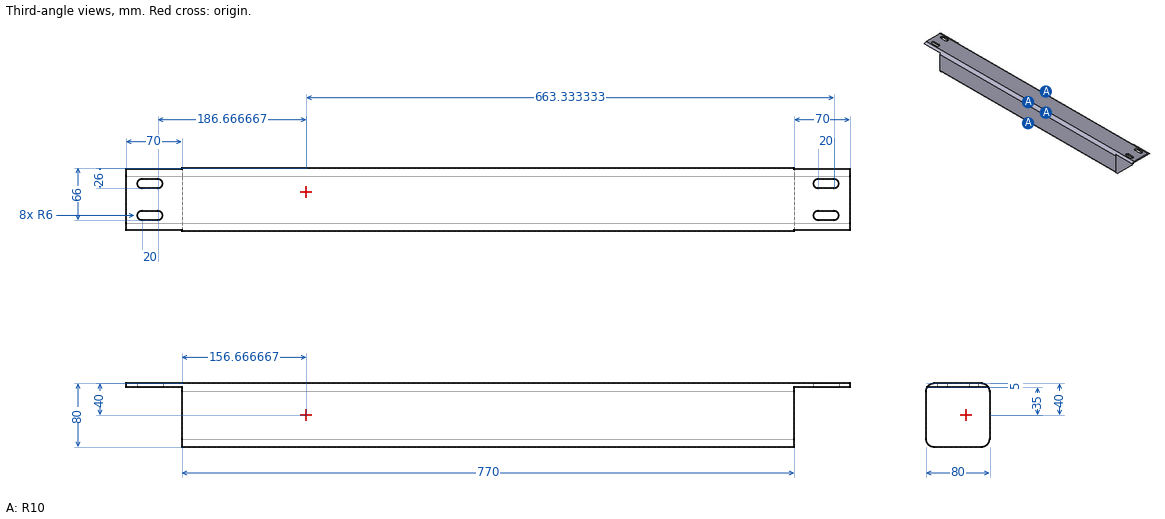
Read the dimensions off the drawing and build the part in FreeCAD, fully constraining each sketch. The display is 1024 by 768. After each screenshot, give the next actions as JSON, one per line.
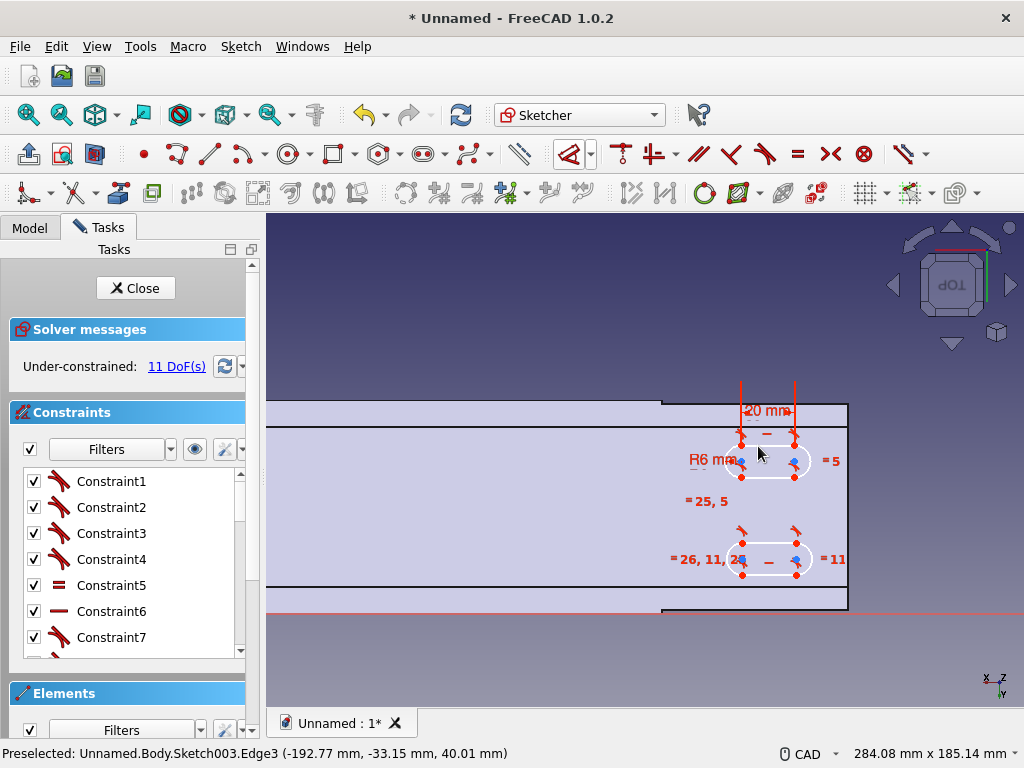
{"action": "left_click", "coordinate": [759, 543]}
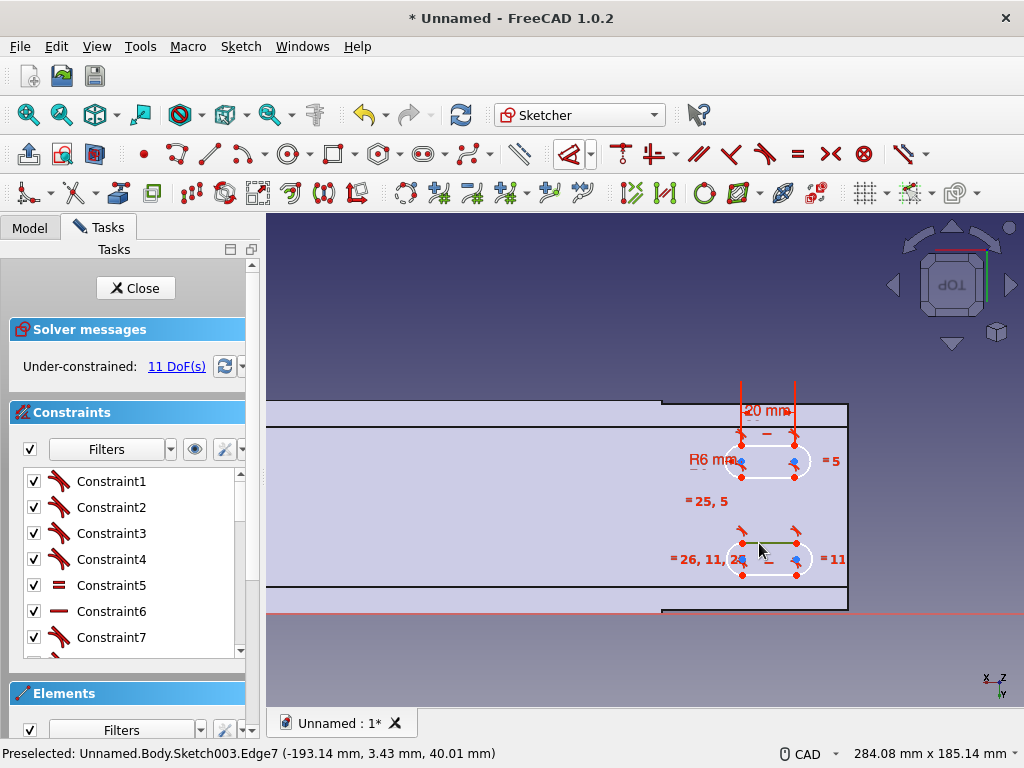
{"action": "left_click", "coordinate": [590, 154]}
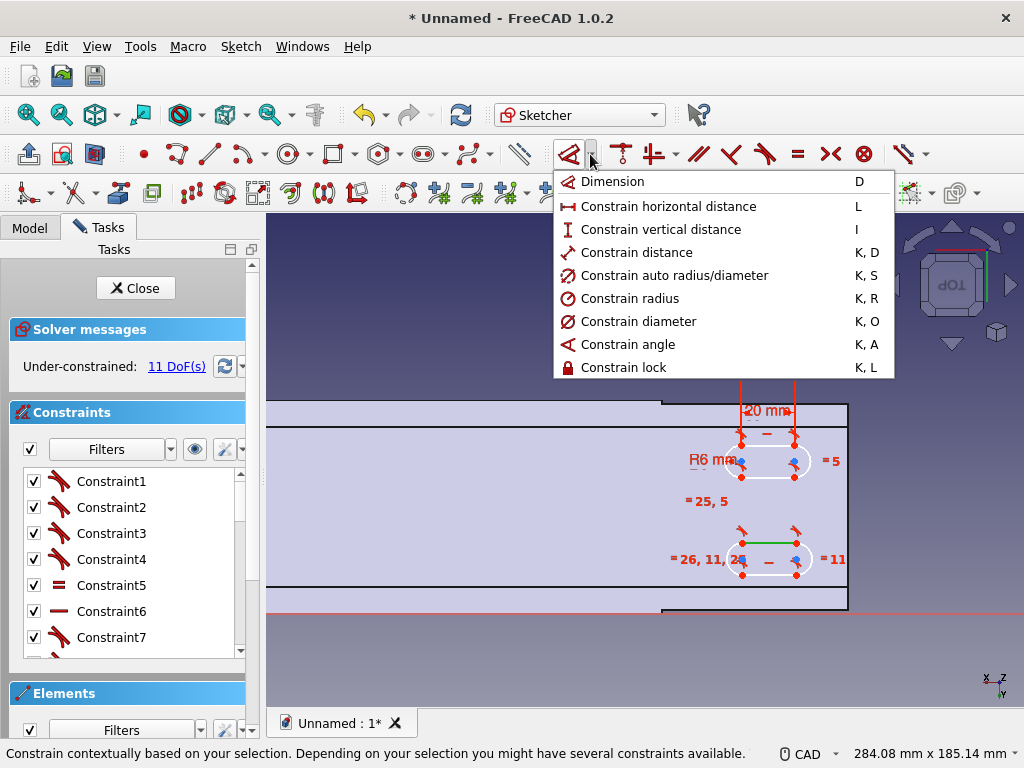
{"action": "left_click", "coordinate": [724, 206]}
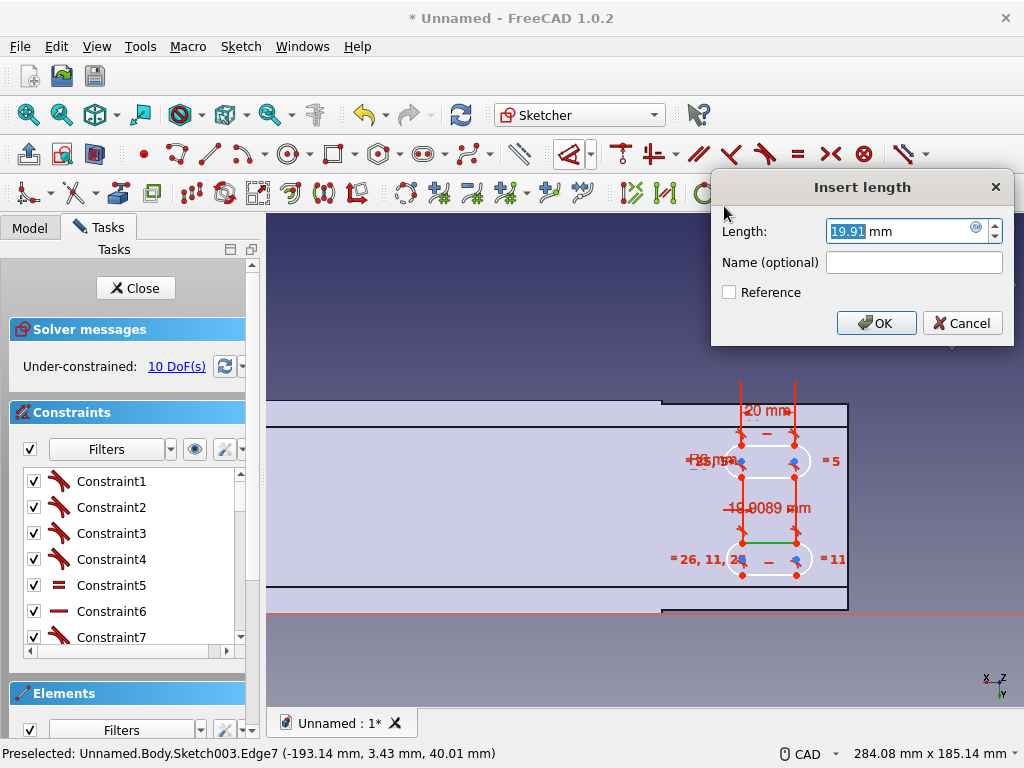
{"action": "type", "text": "20"}
{"action": "key", "text": "Return"}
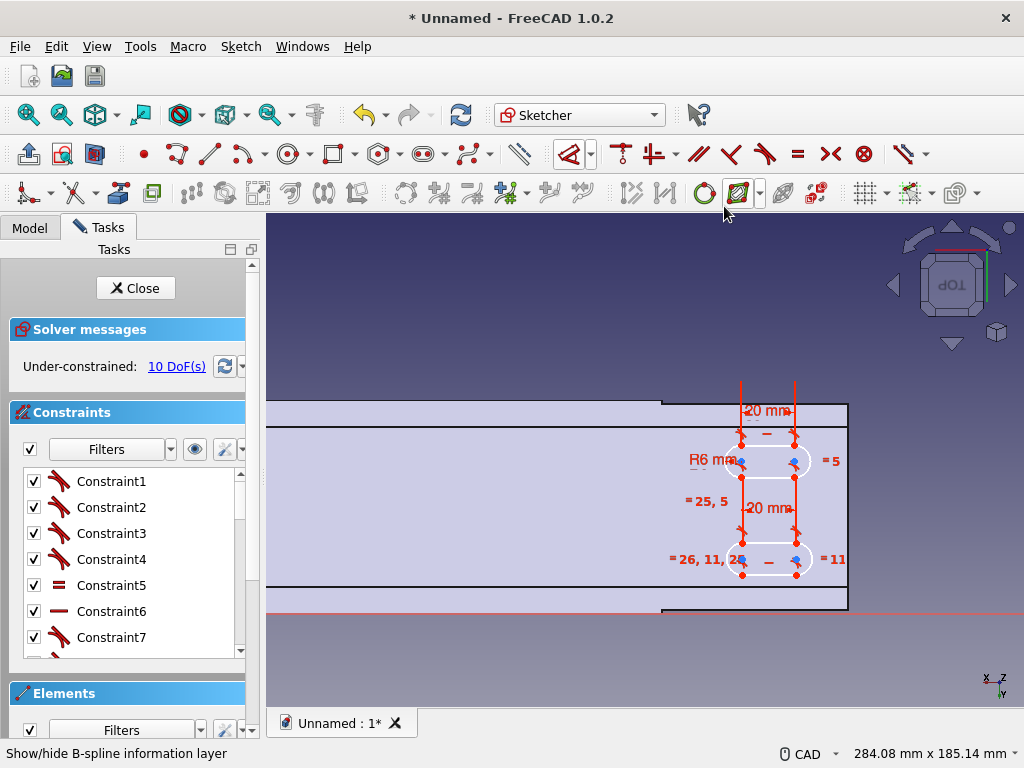
{"action": "scroll", "coordinate": [763, 447], "scroll_direction": "down", "scroll_amount": 9}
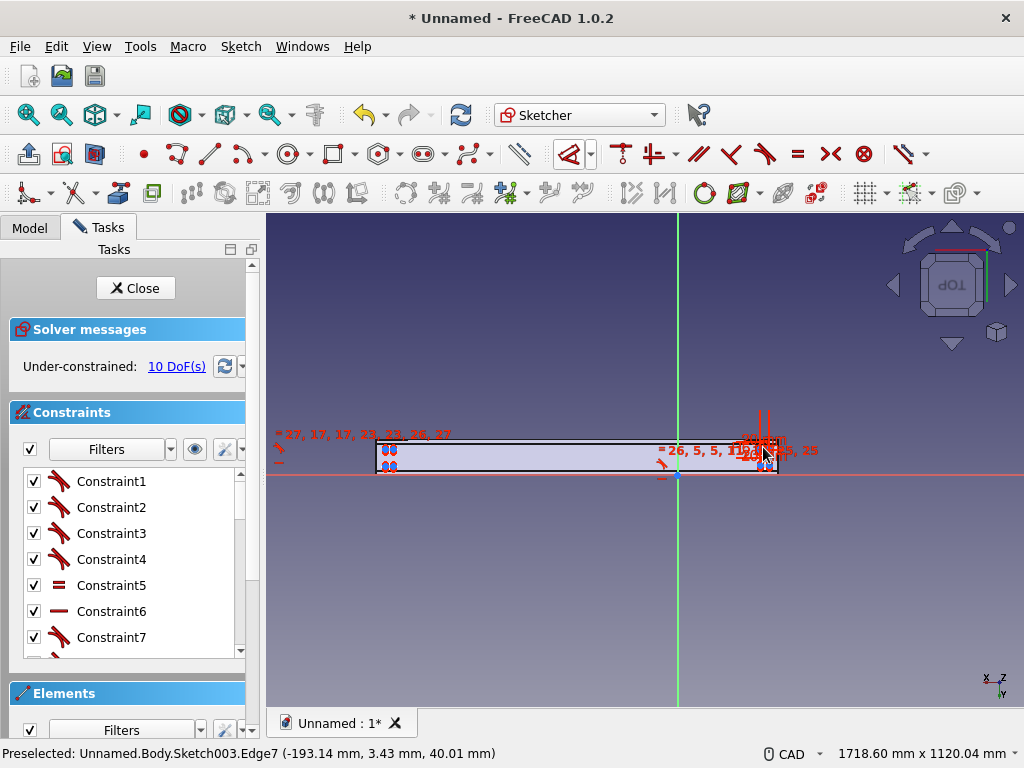
{"action": "scroll", "coordinate": [388, 464], "scroll_direction": "up", "scroll_amount": 9}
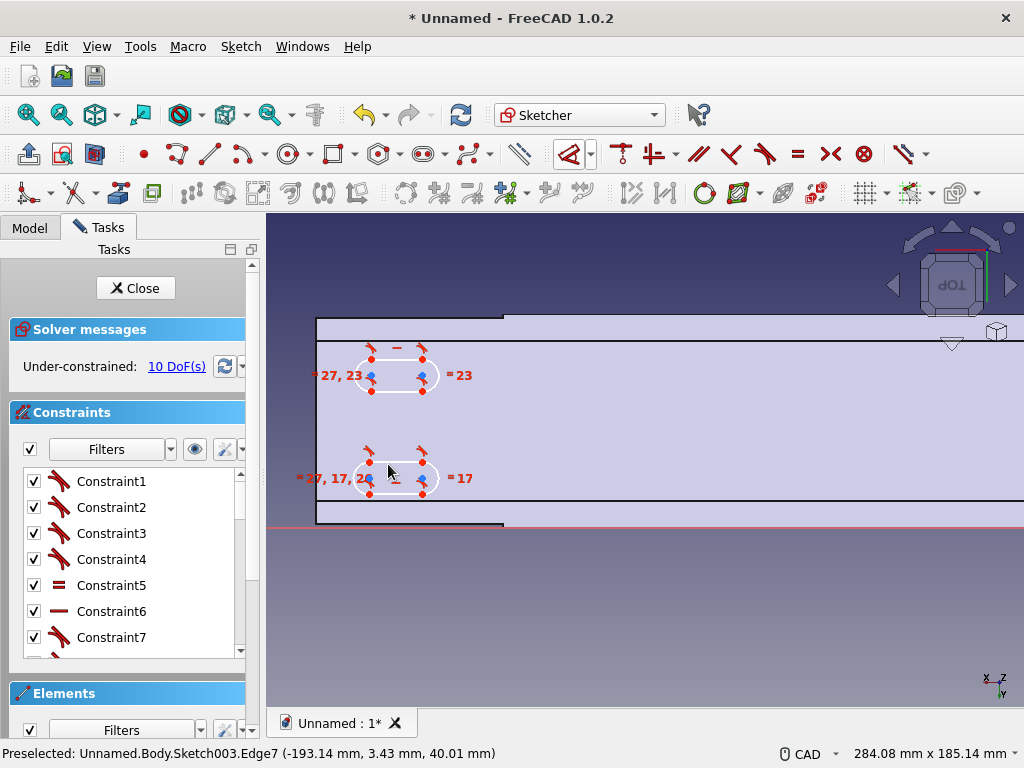
{"action": "left_click", "coordinate": [385, 462]}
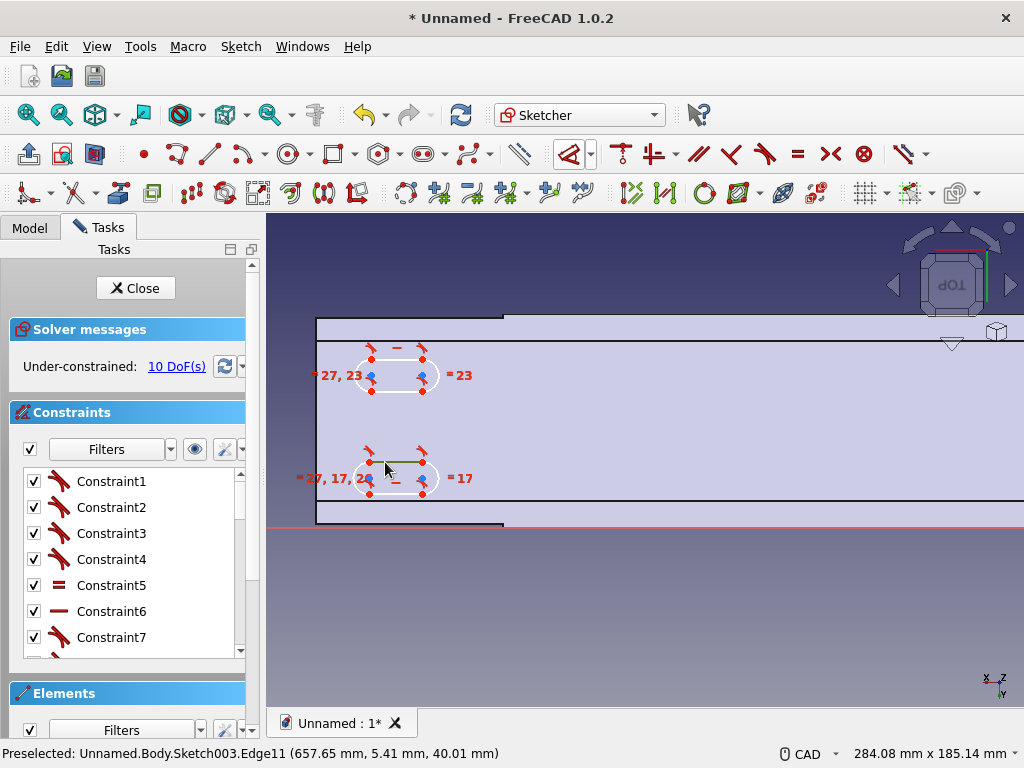
{"action": "key", "text": "l"}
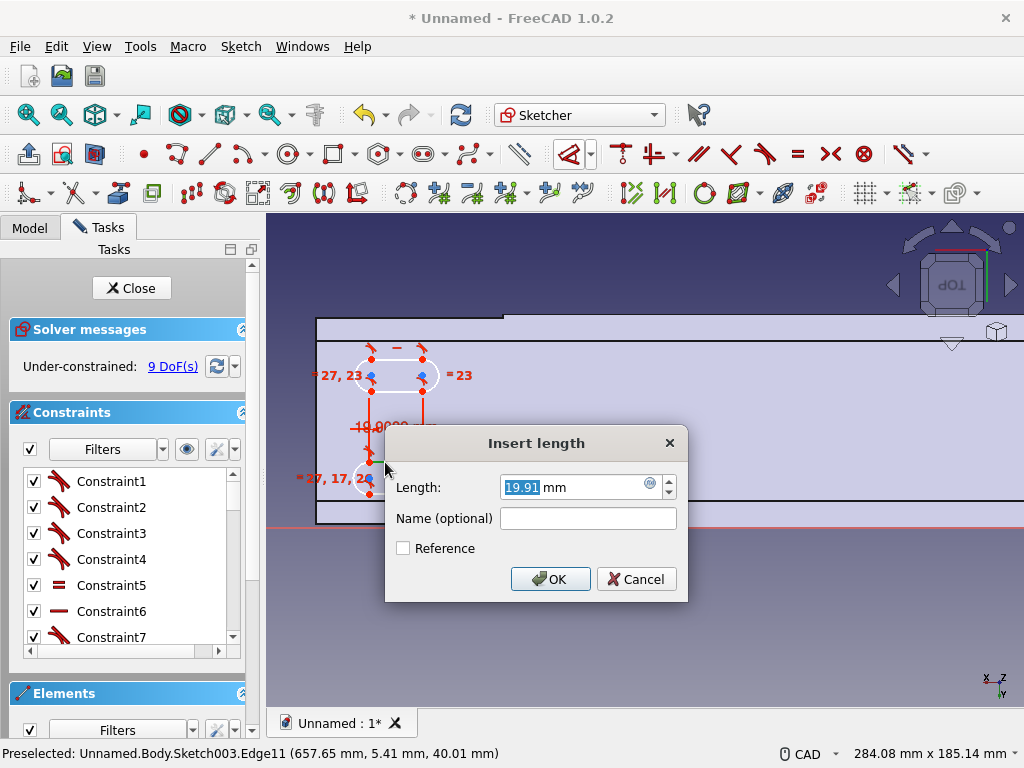
{"action": "type", "text": "20"}
{"action": "key", "text": "Return"}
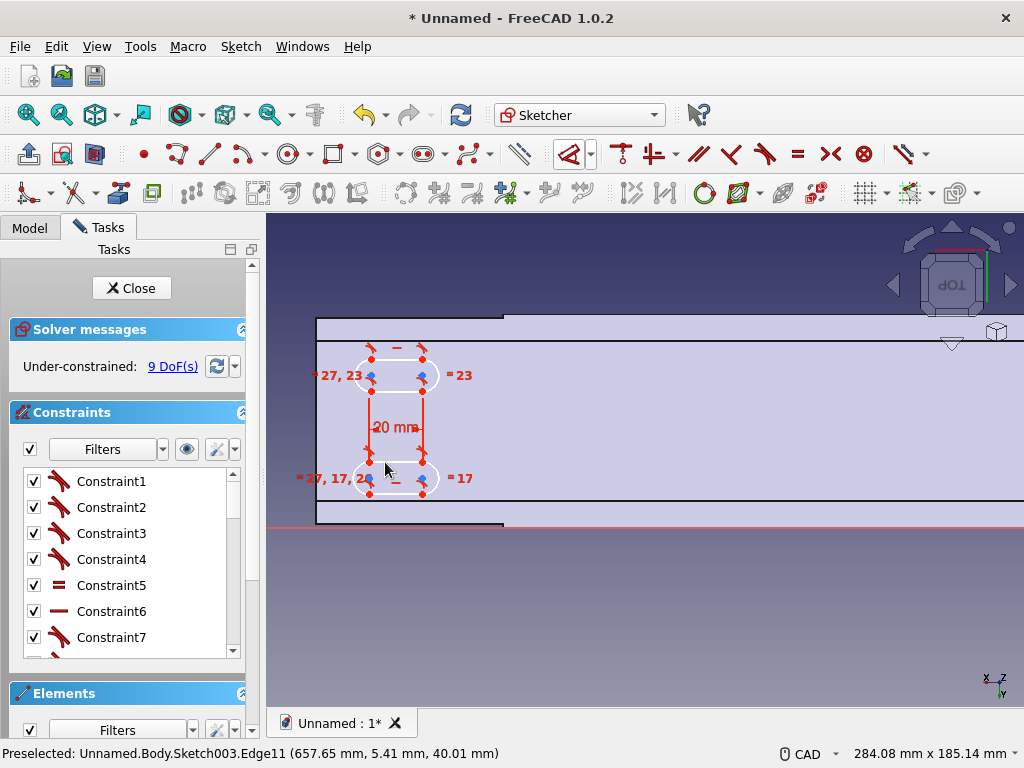
{"action": "left_click", "coordinate": [387, 360]}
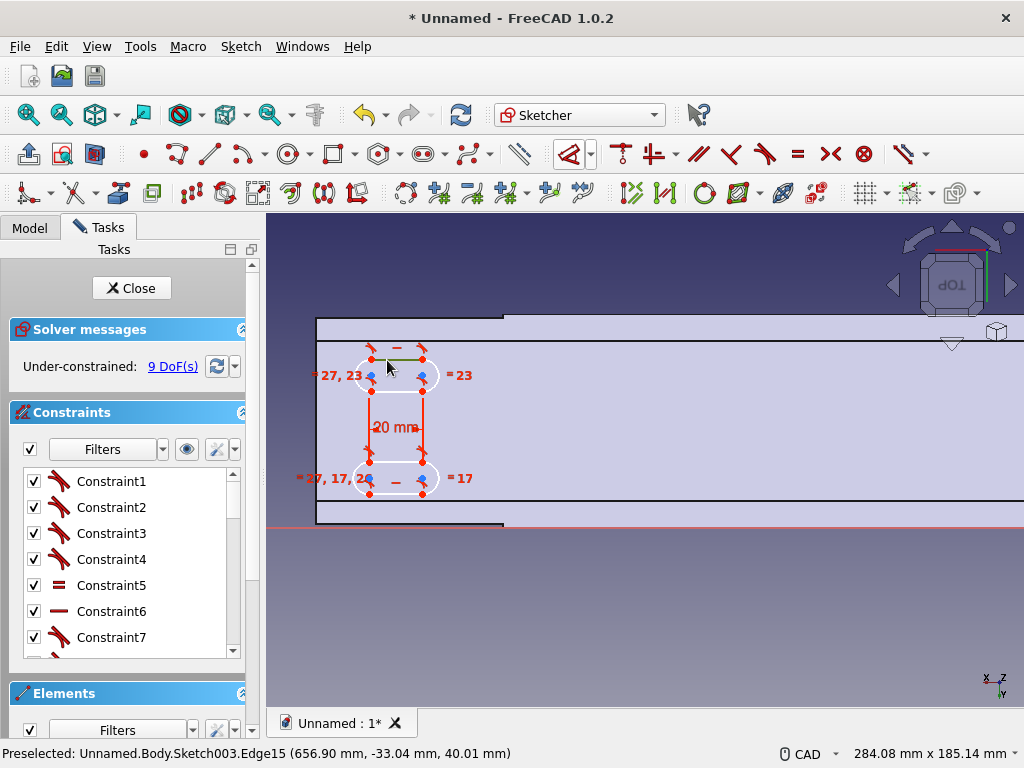
{"action": "left_click", "coordinate": [590, 154]}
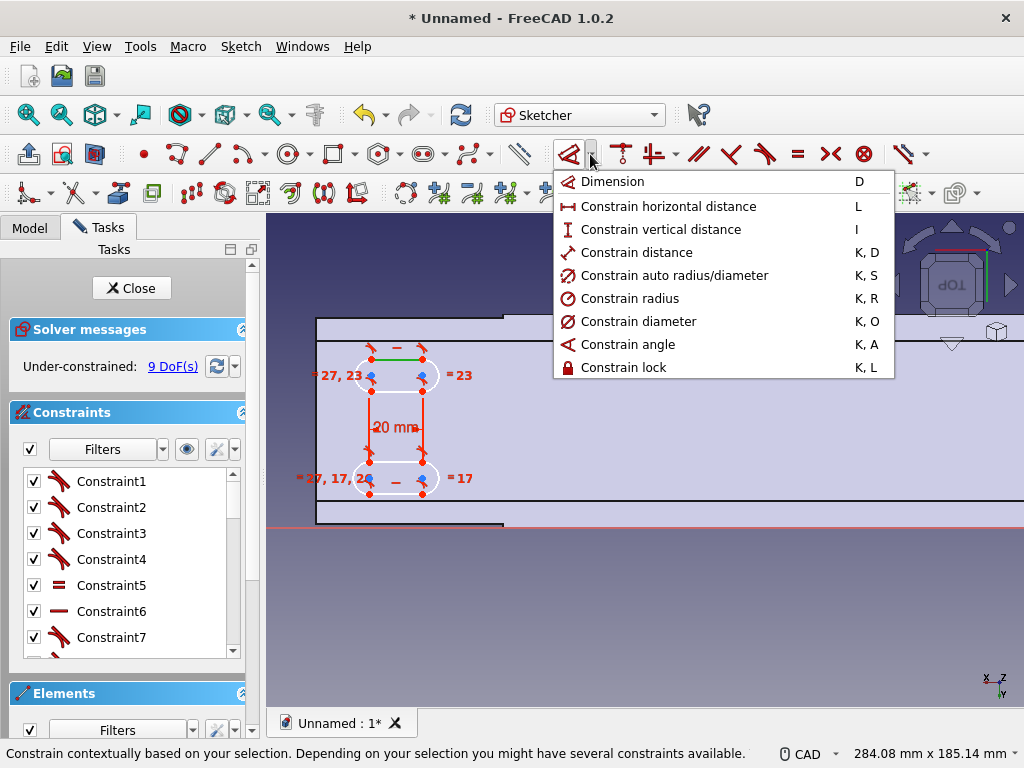
{"action": "left_click", "coordinate": [724, 206]}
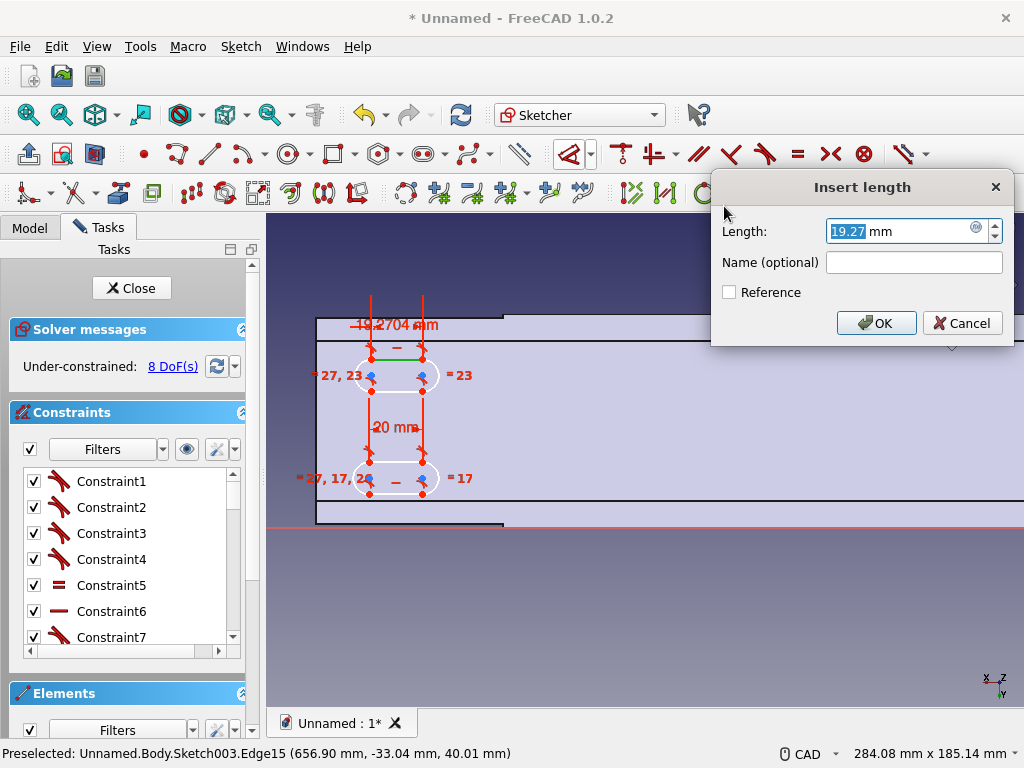
{"action": "type", "text": "20"}
{"action": "key", "text": "Return"}